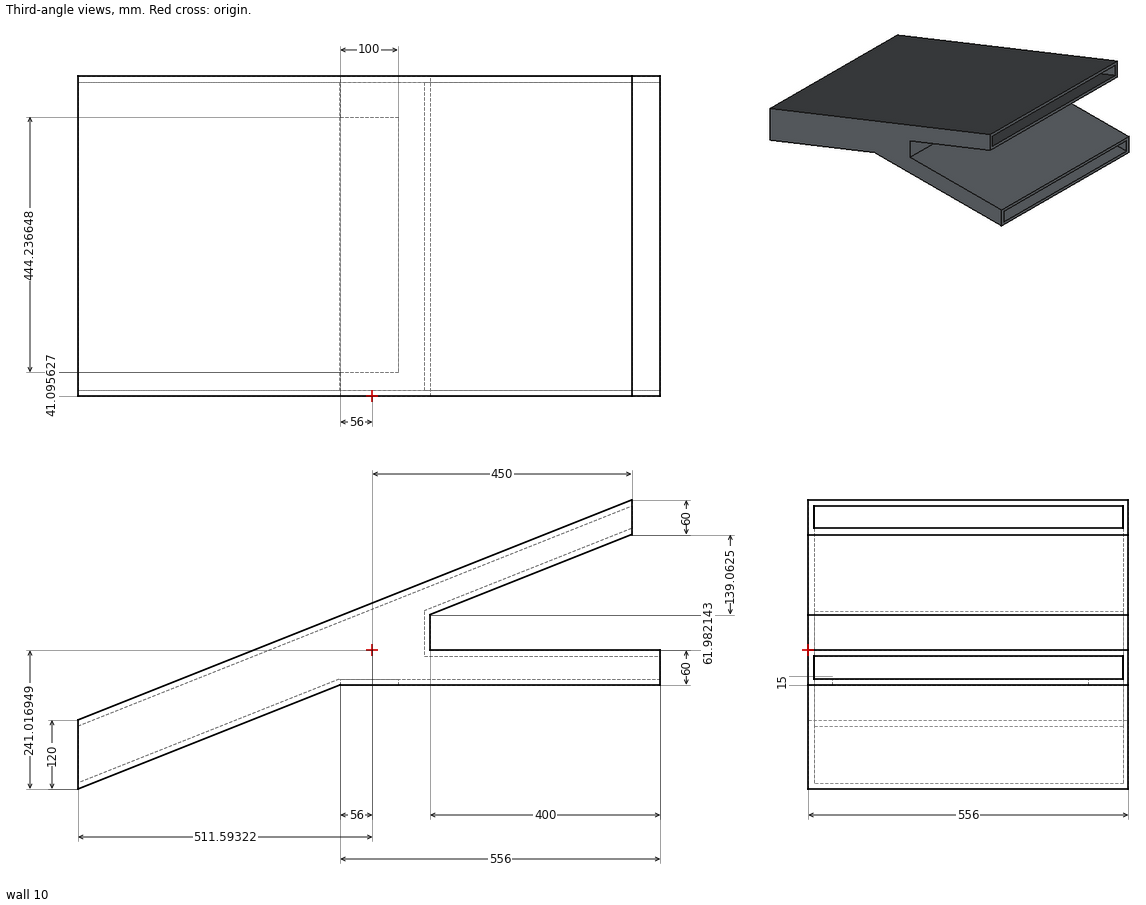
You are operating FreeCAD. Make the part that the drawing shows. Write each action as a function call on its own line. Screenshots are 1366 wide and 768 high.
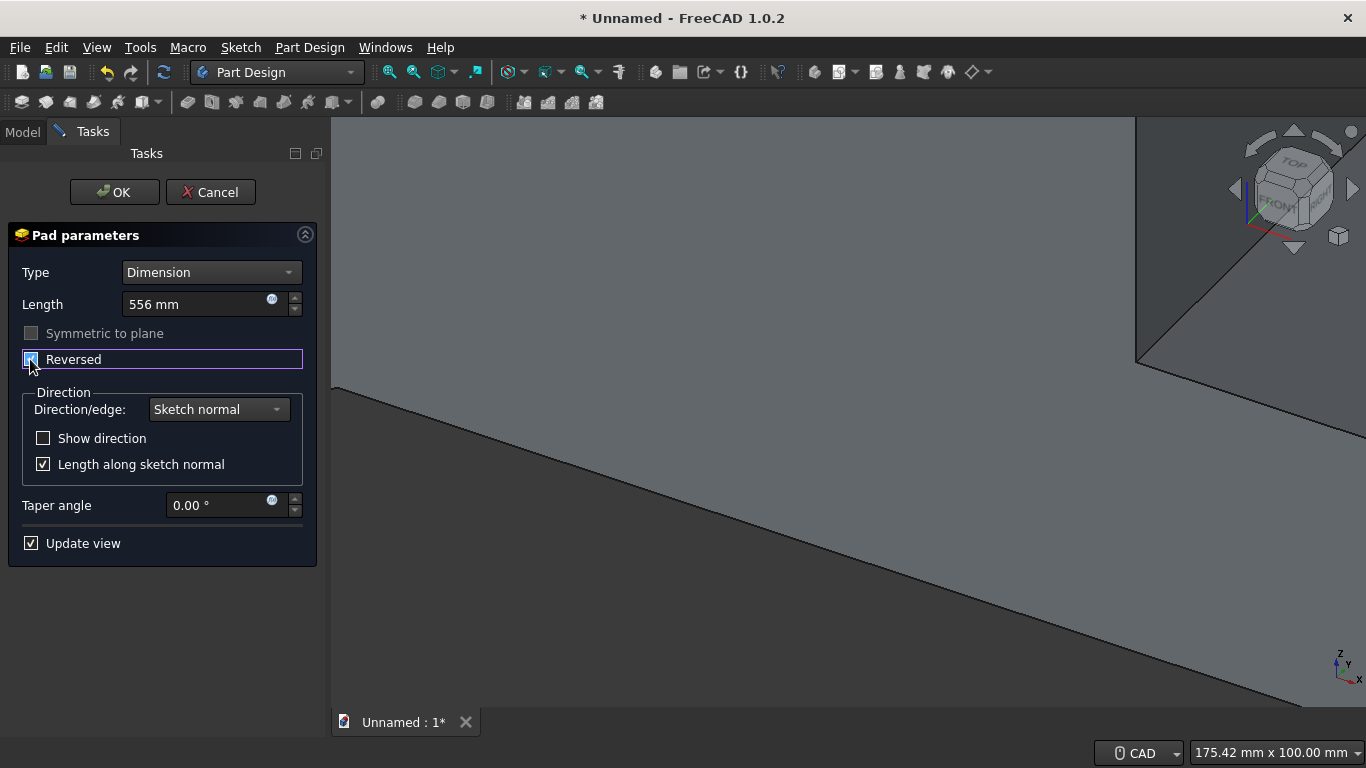
click(115, 192)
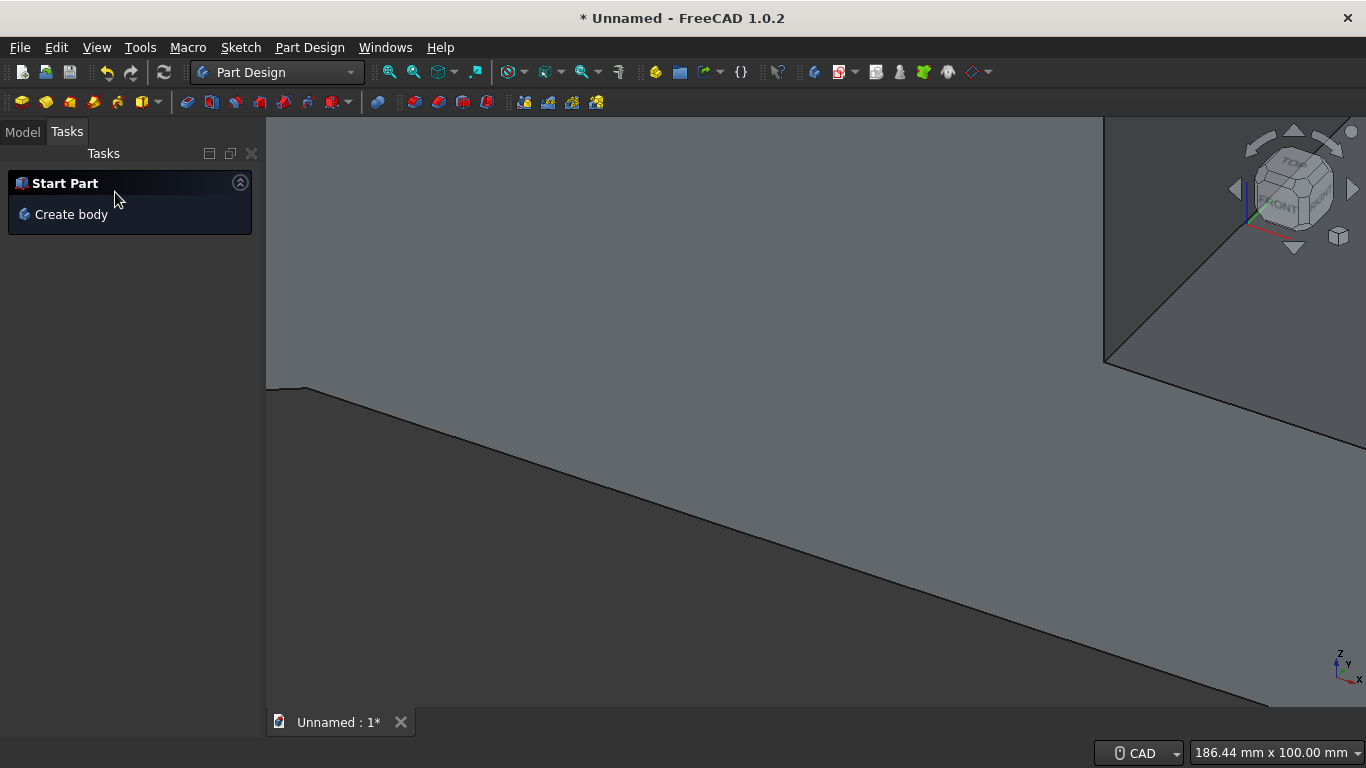
click(390, 72)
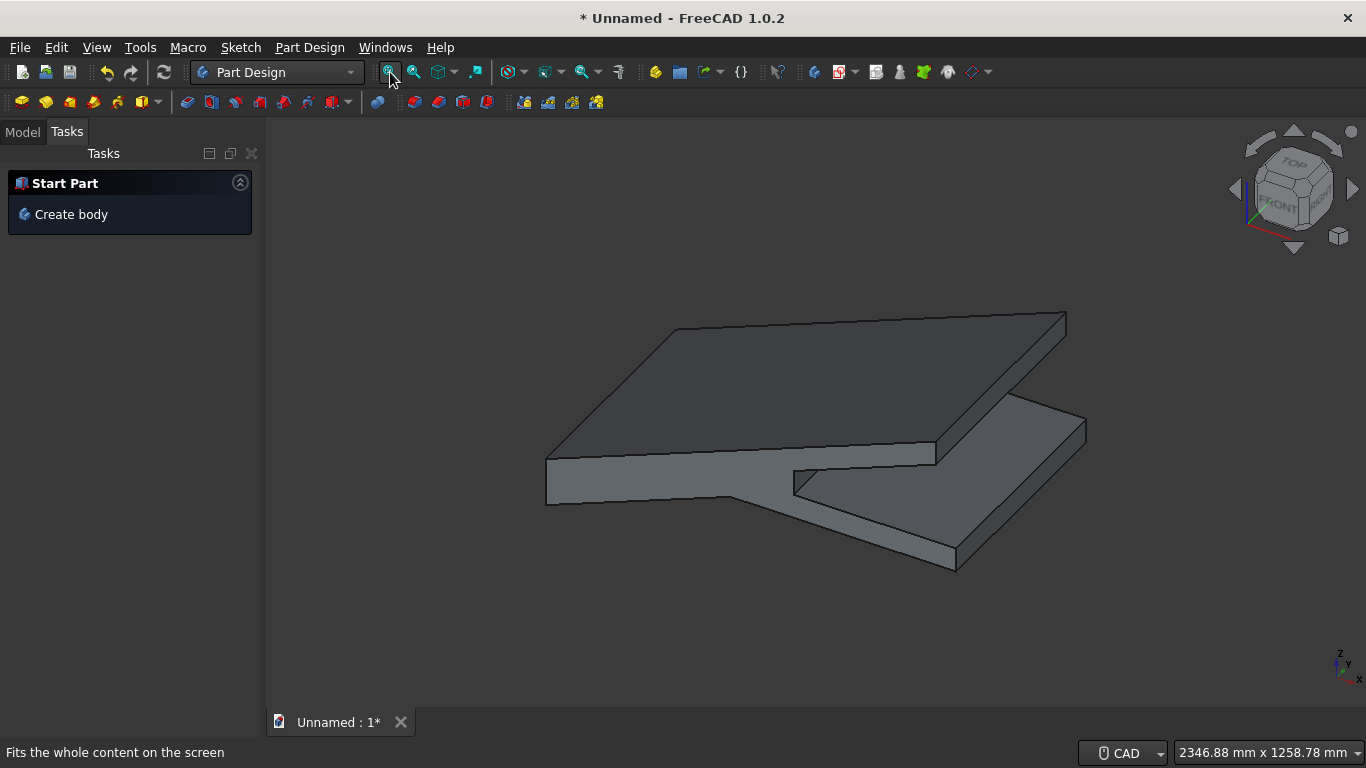
click(1057, 335)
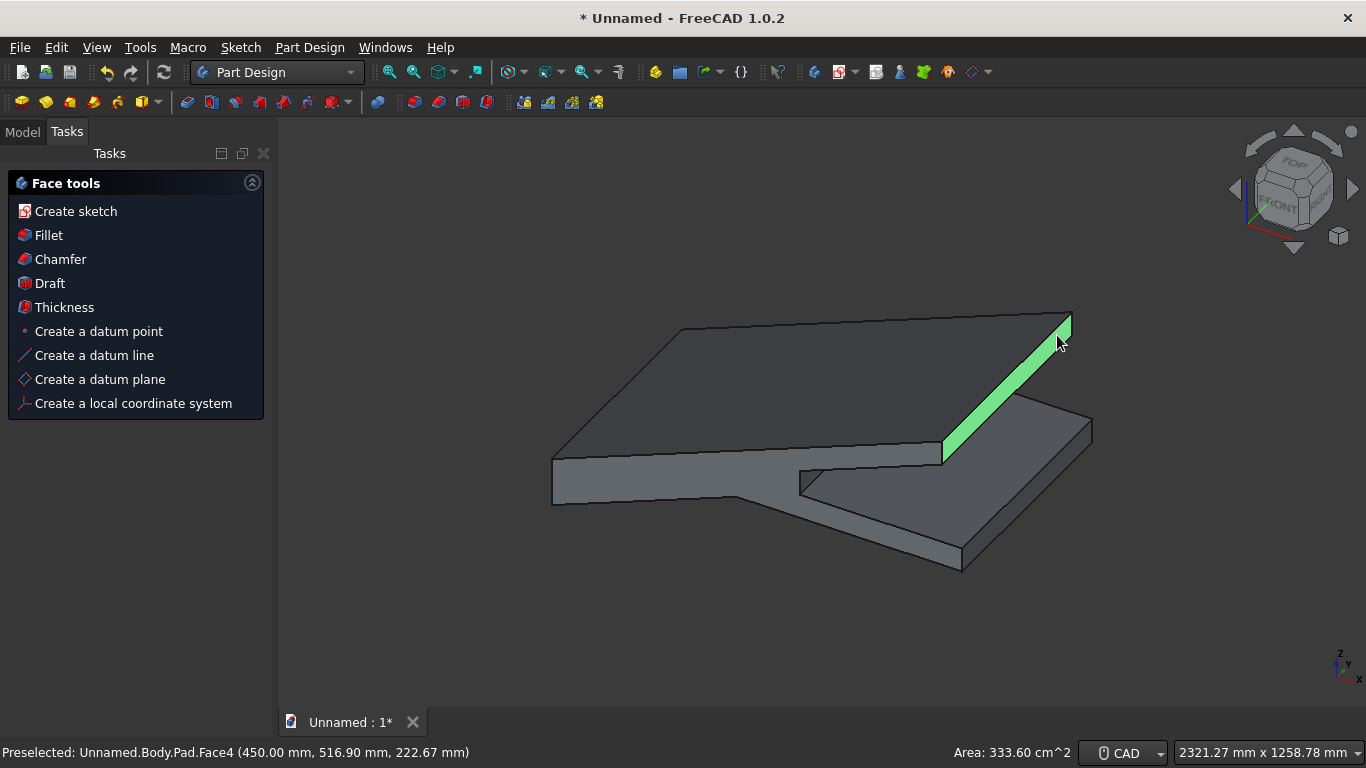
click(1065, 461, ctrl)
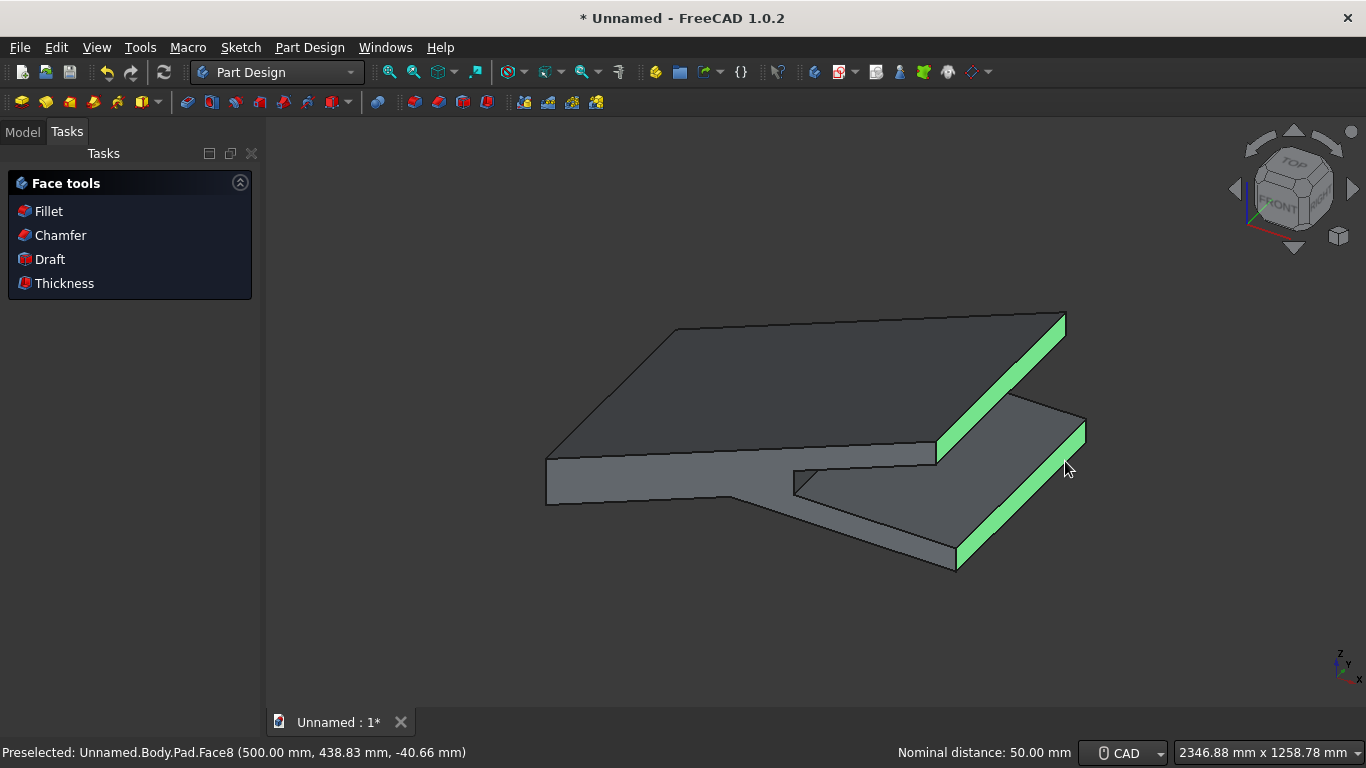
key(0)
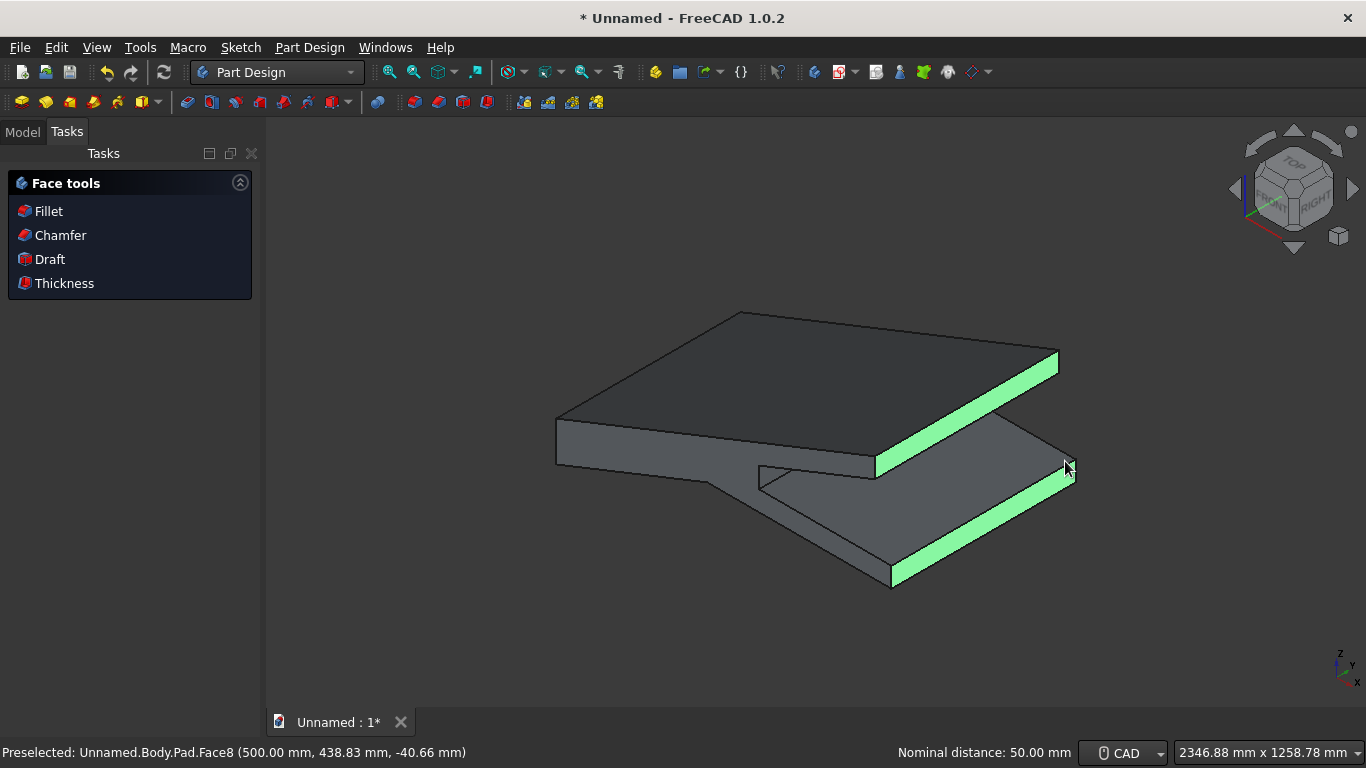
key(2)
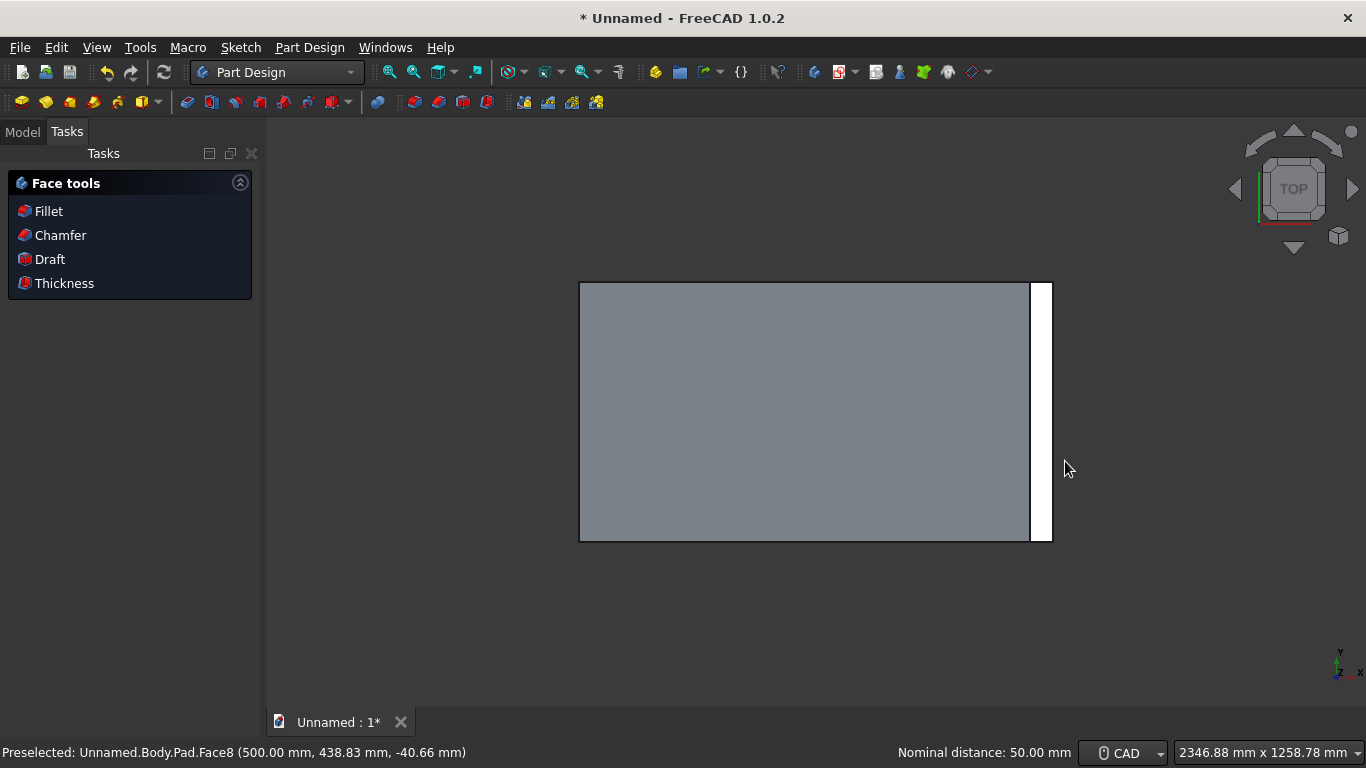
click(390, 72)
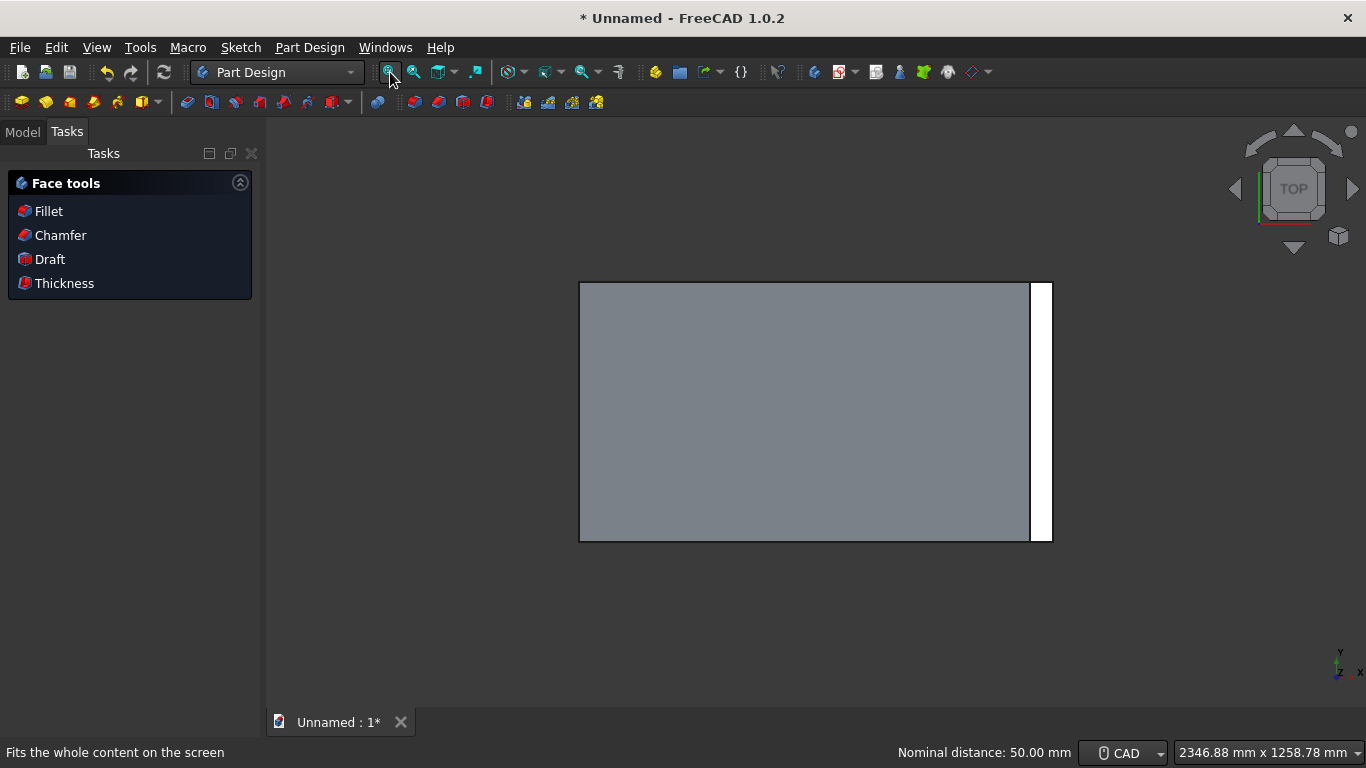
key(1)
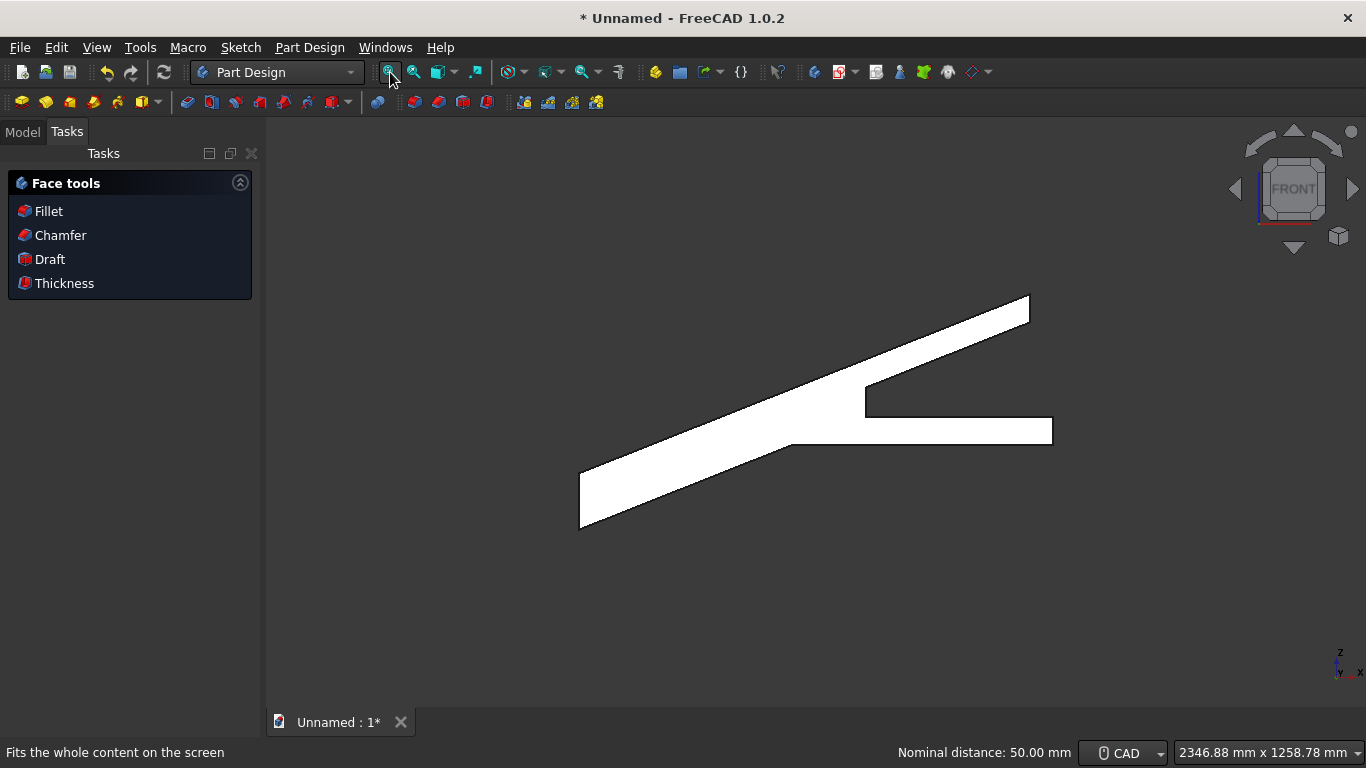
click(390, 72)